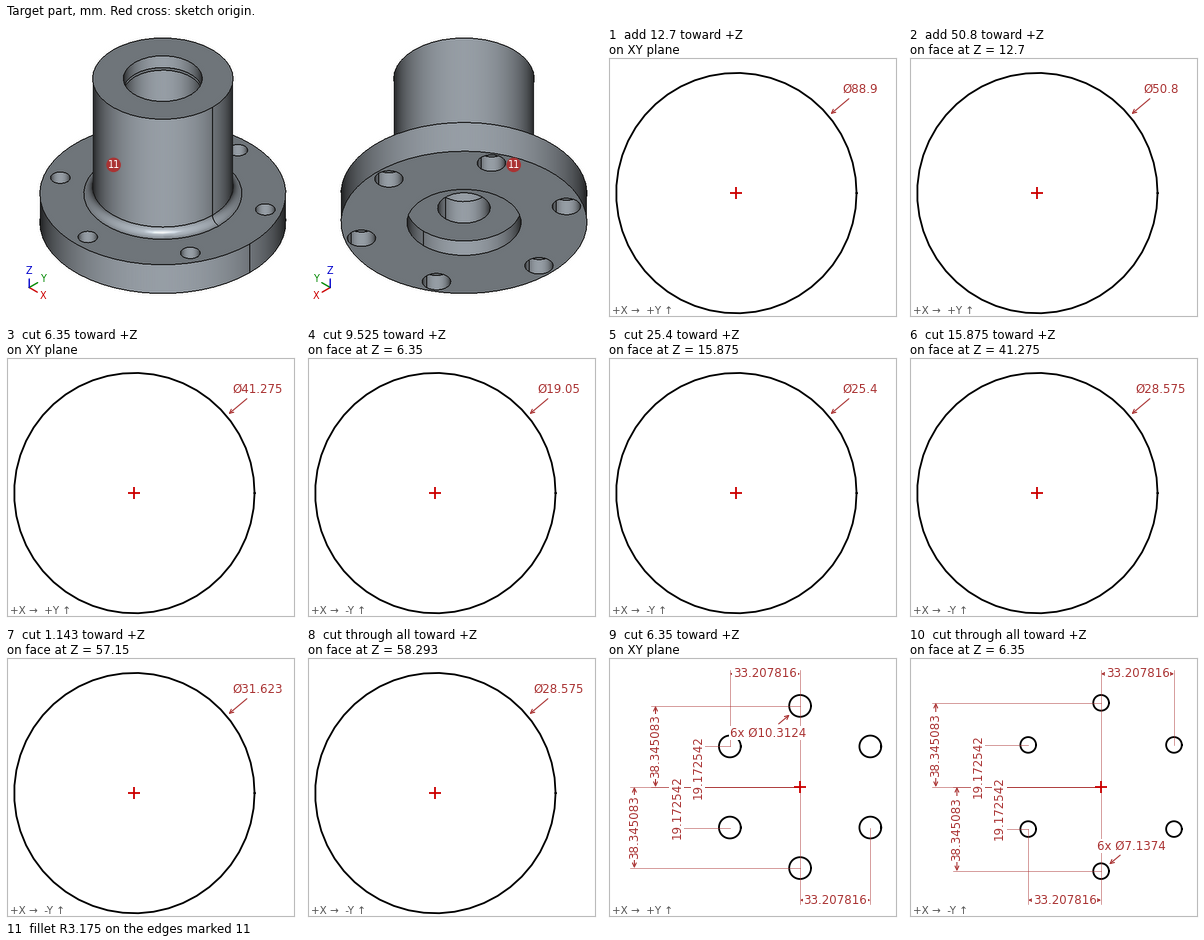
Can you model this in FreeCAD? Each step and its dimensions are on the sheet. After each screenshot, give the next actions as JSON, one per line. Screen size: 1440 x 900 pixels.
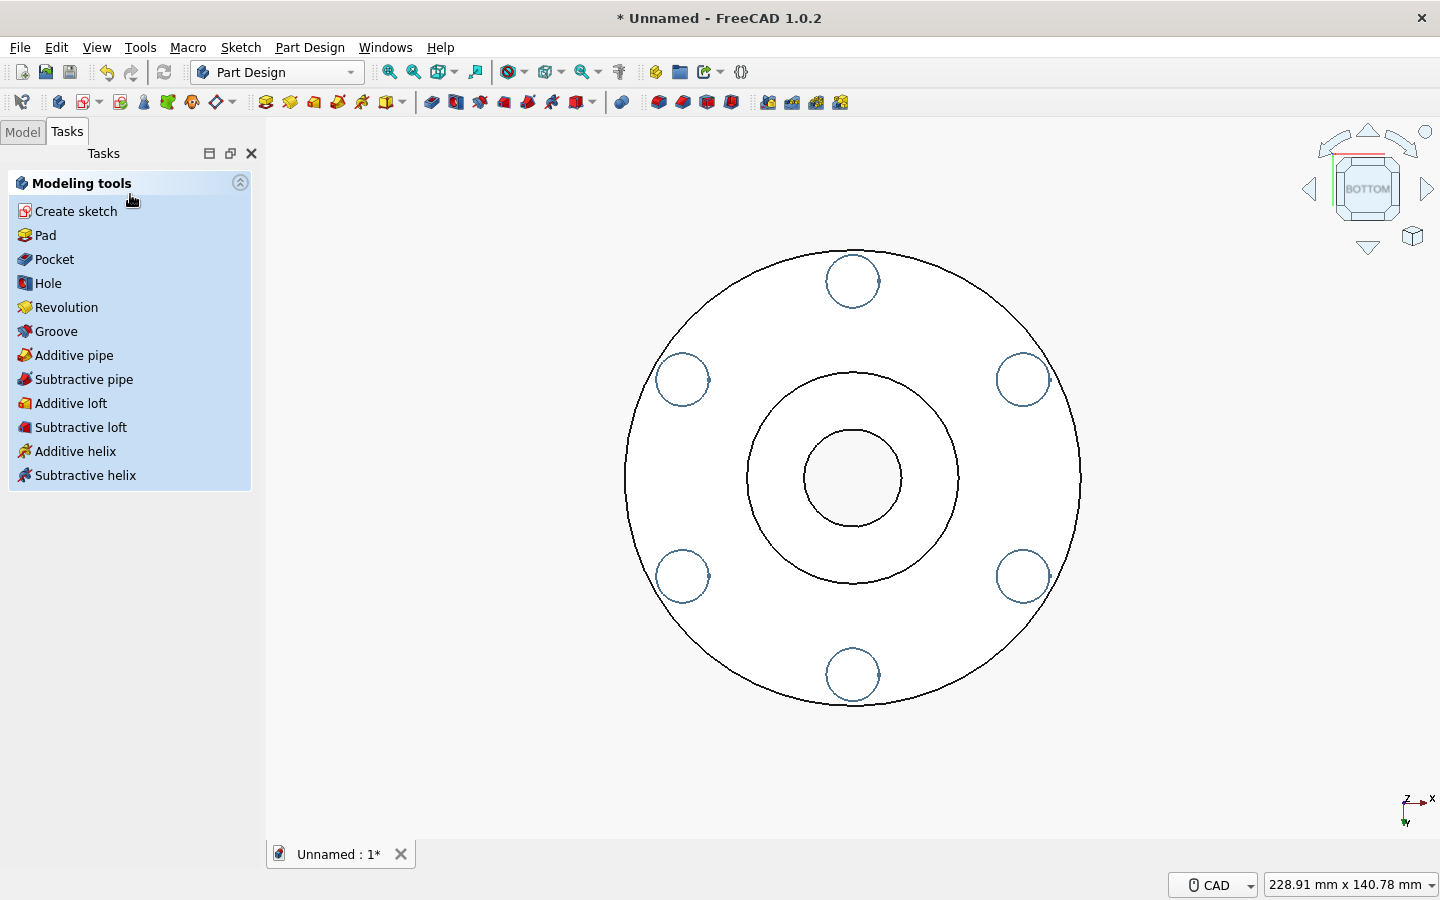
{"action": "left_click", "coordinate": [432, 102]}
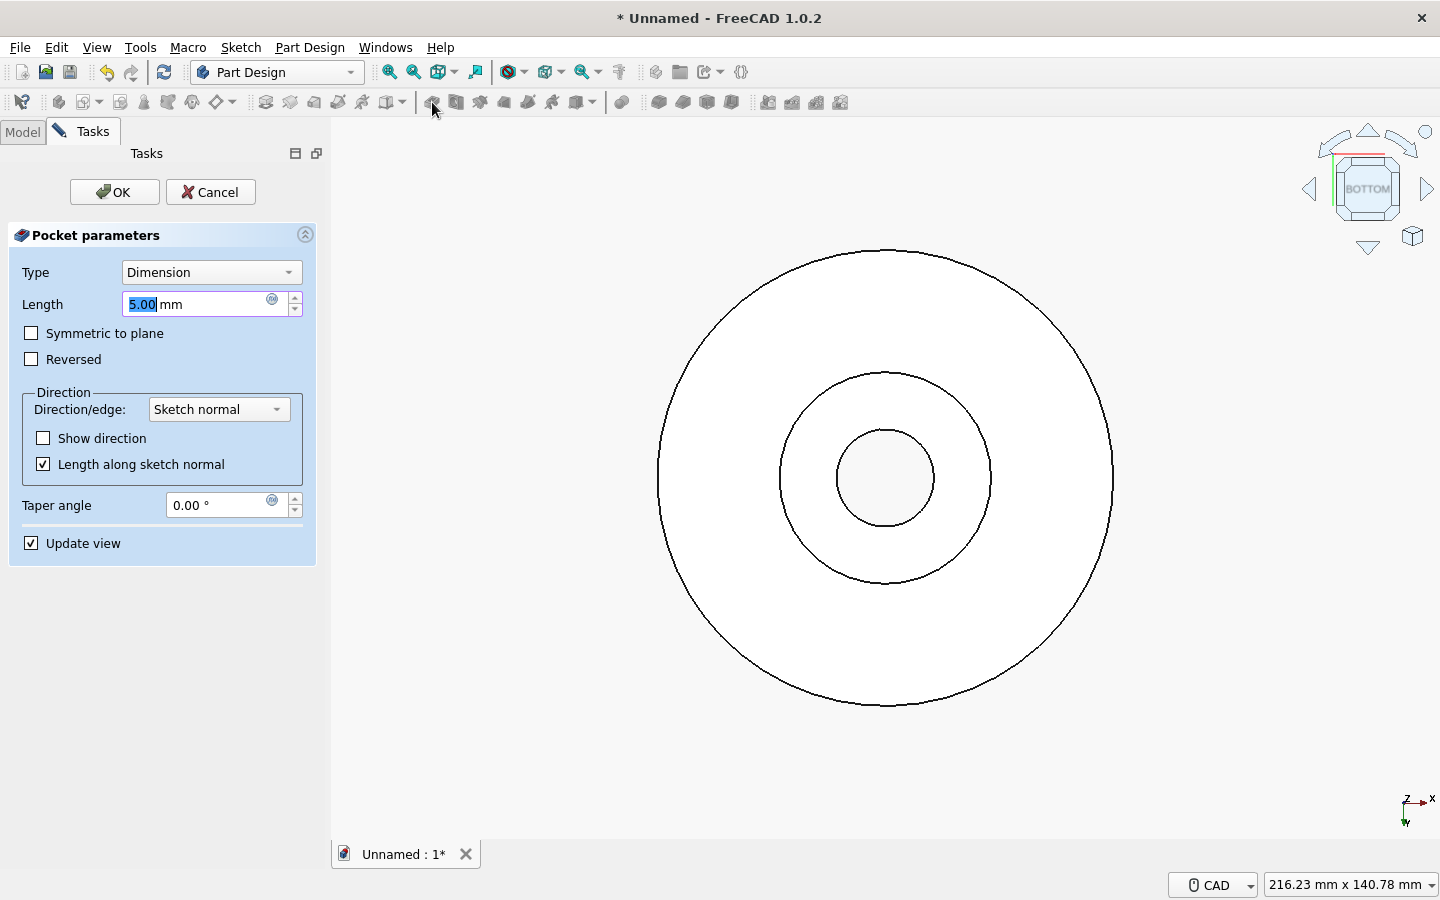
{"action": "type", "text": "6.35"}
{"action": "key", "text": "Tab"}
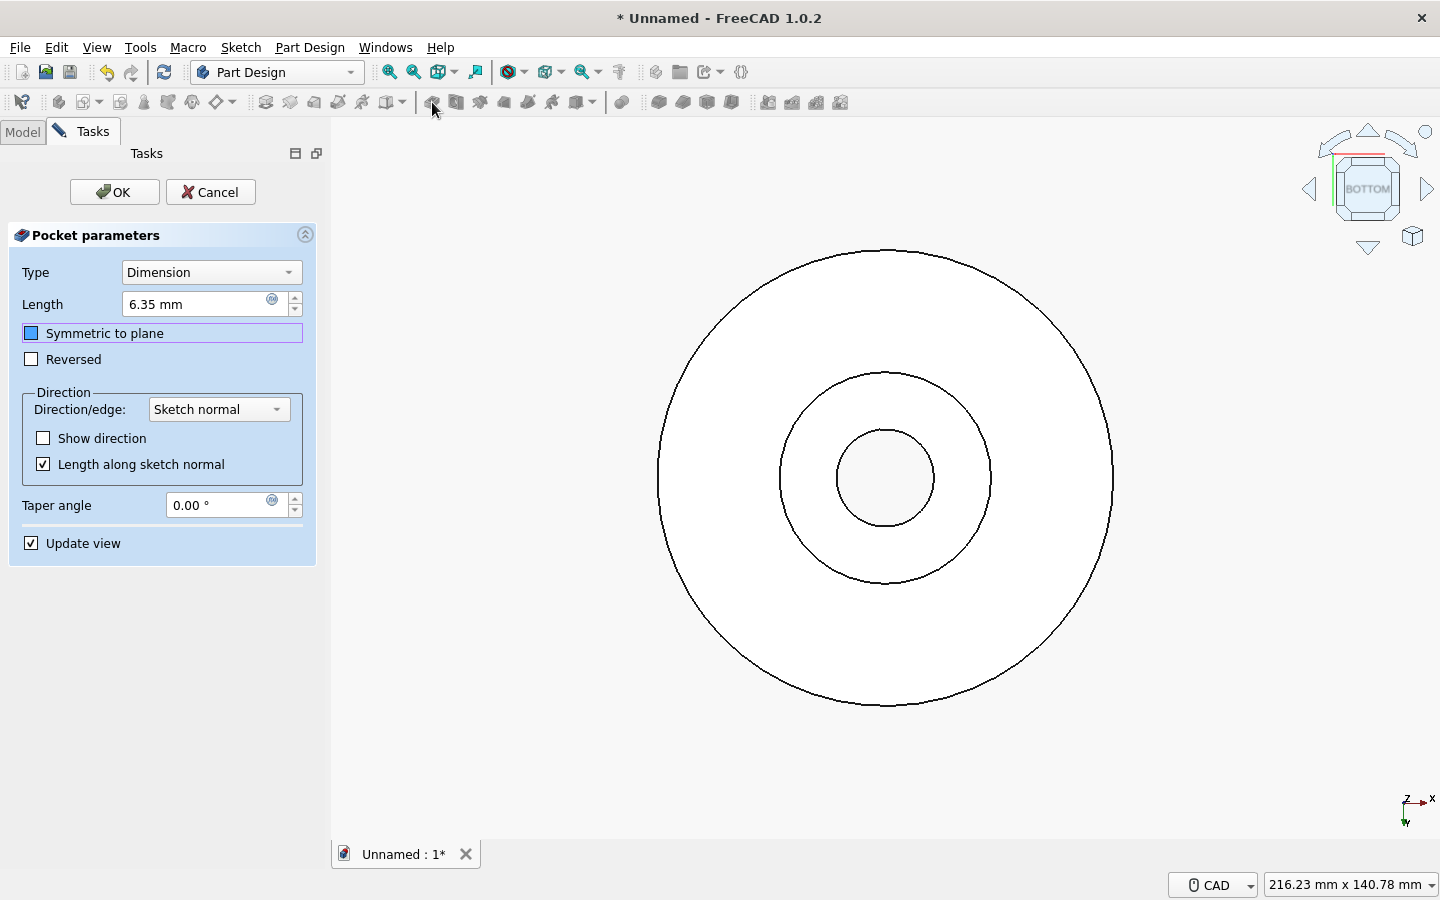
{"action": "left_click", "coordinate": [30, 359]}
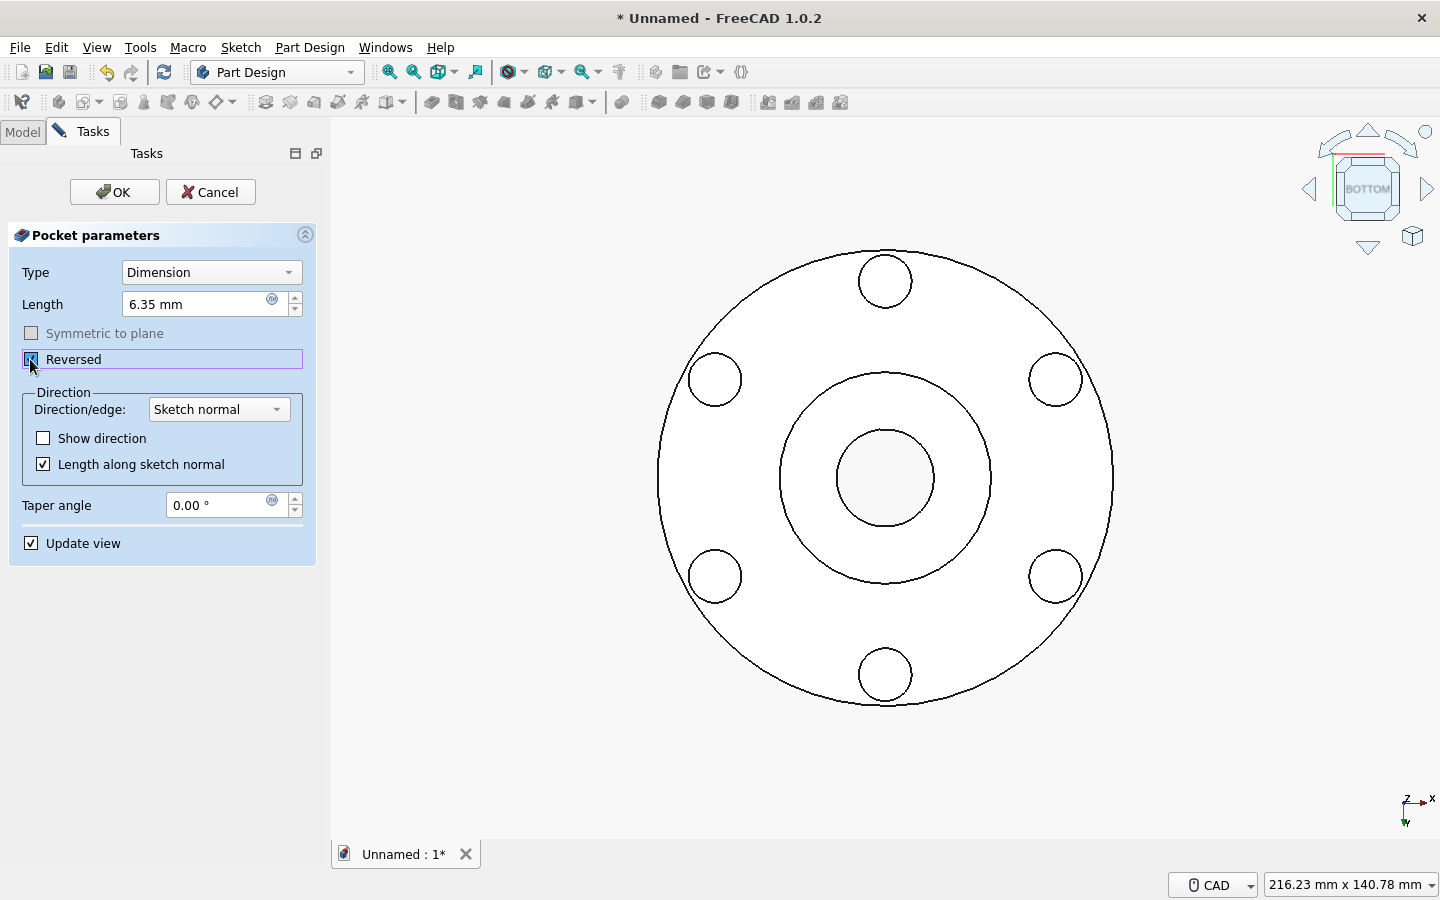
{"action": "left_click", "coordinate": [115, 192]}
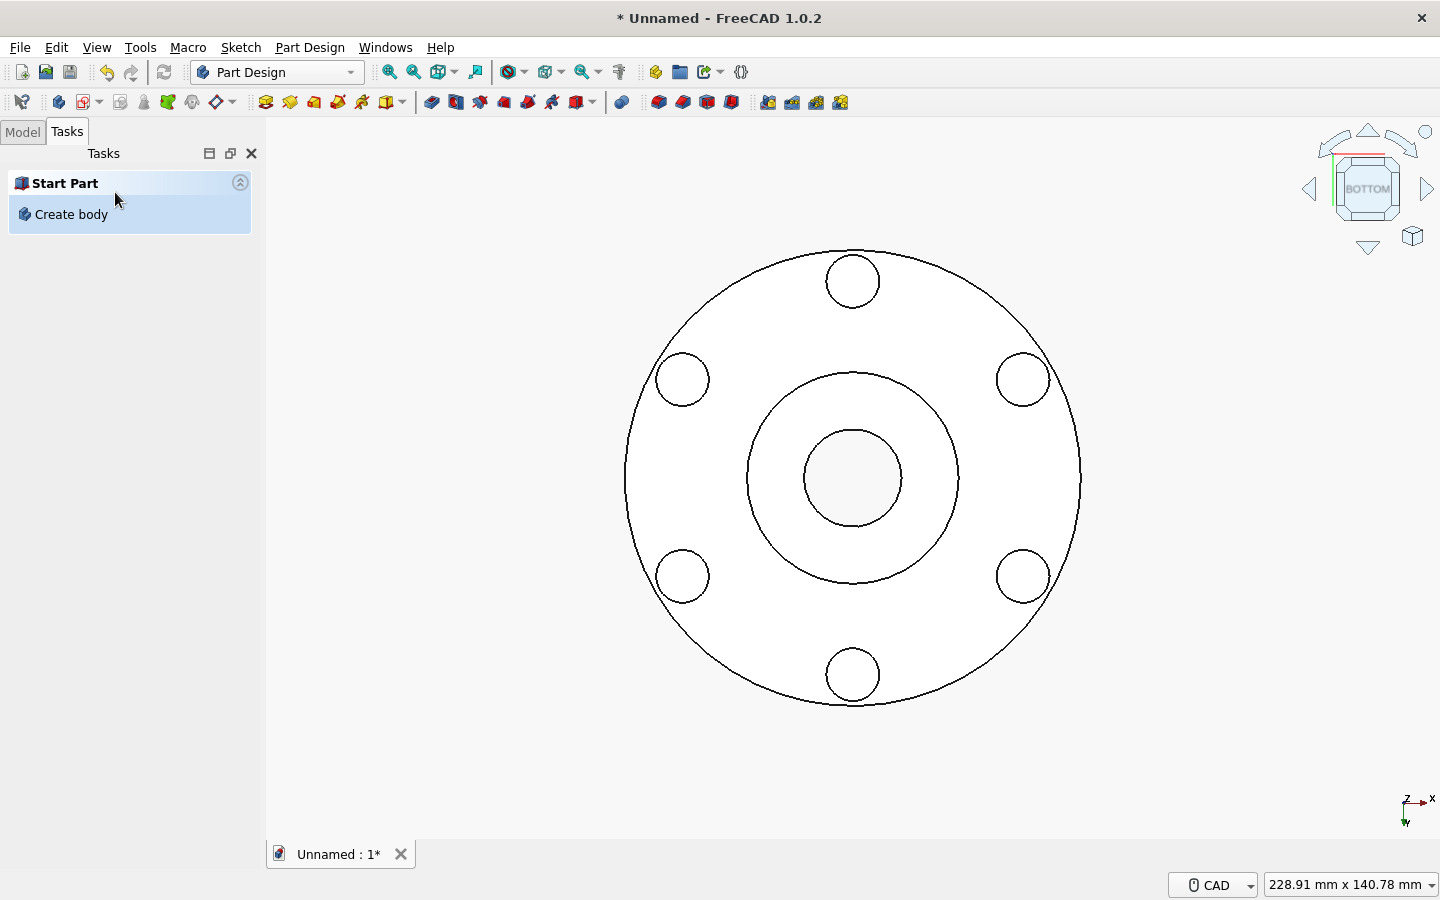
{"action": "left_click", "coordinate": [913, 537]}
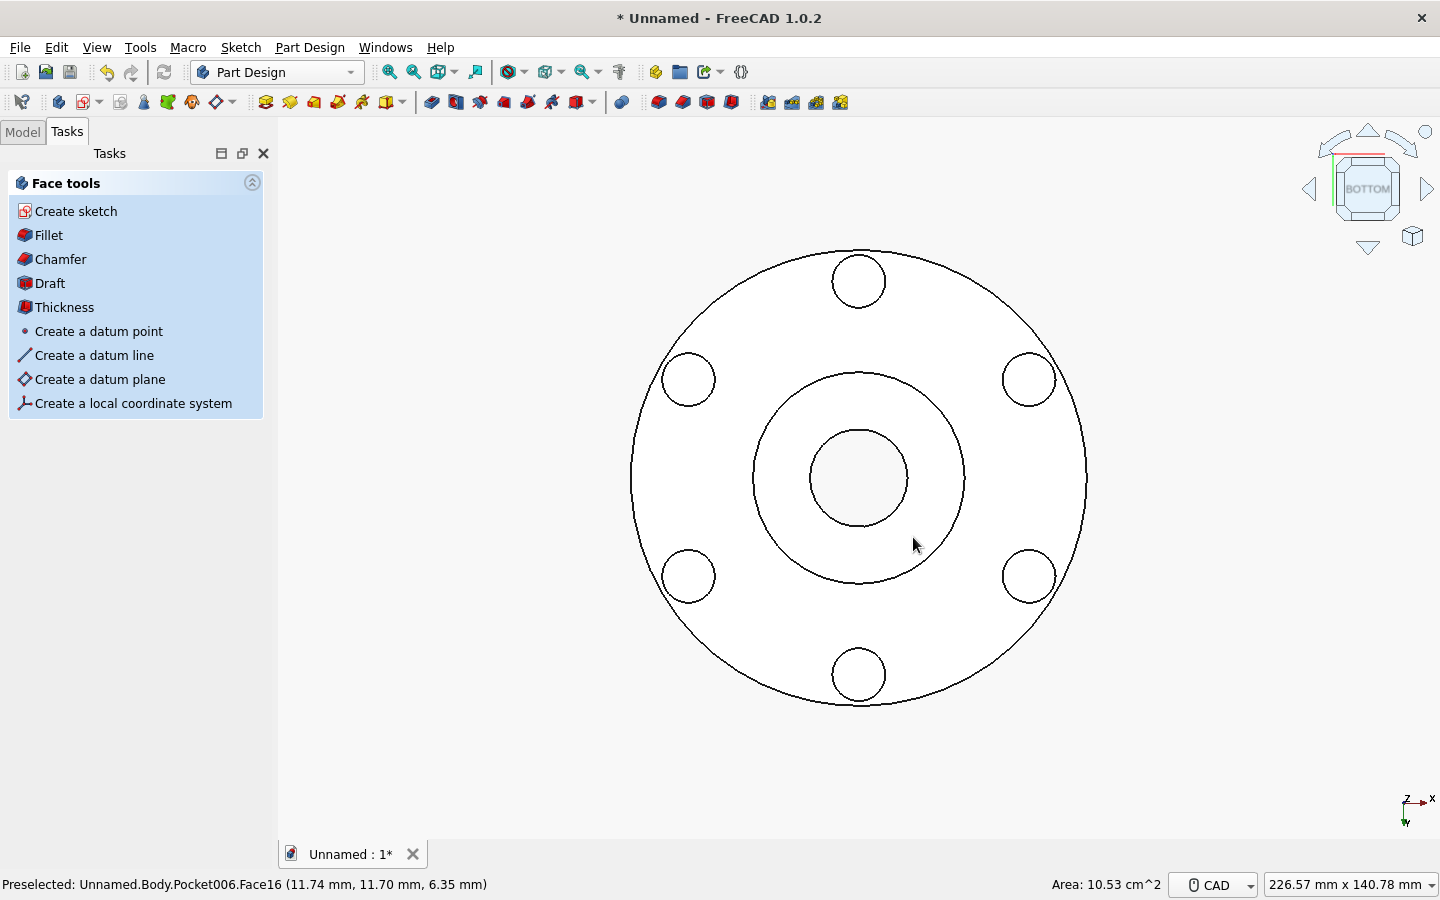
{"action": "left_click", "coordinate": [84, 102]}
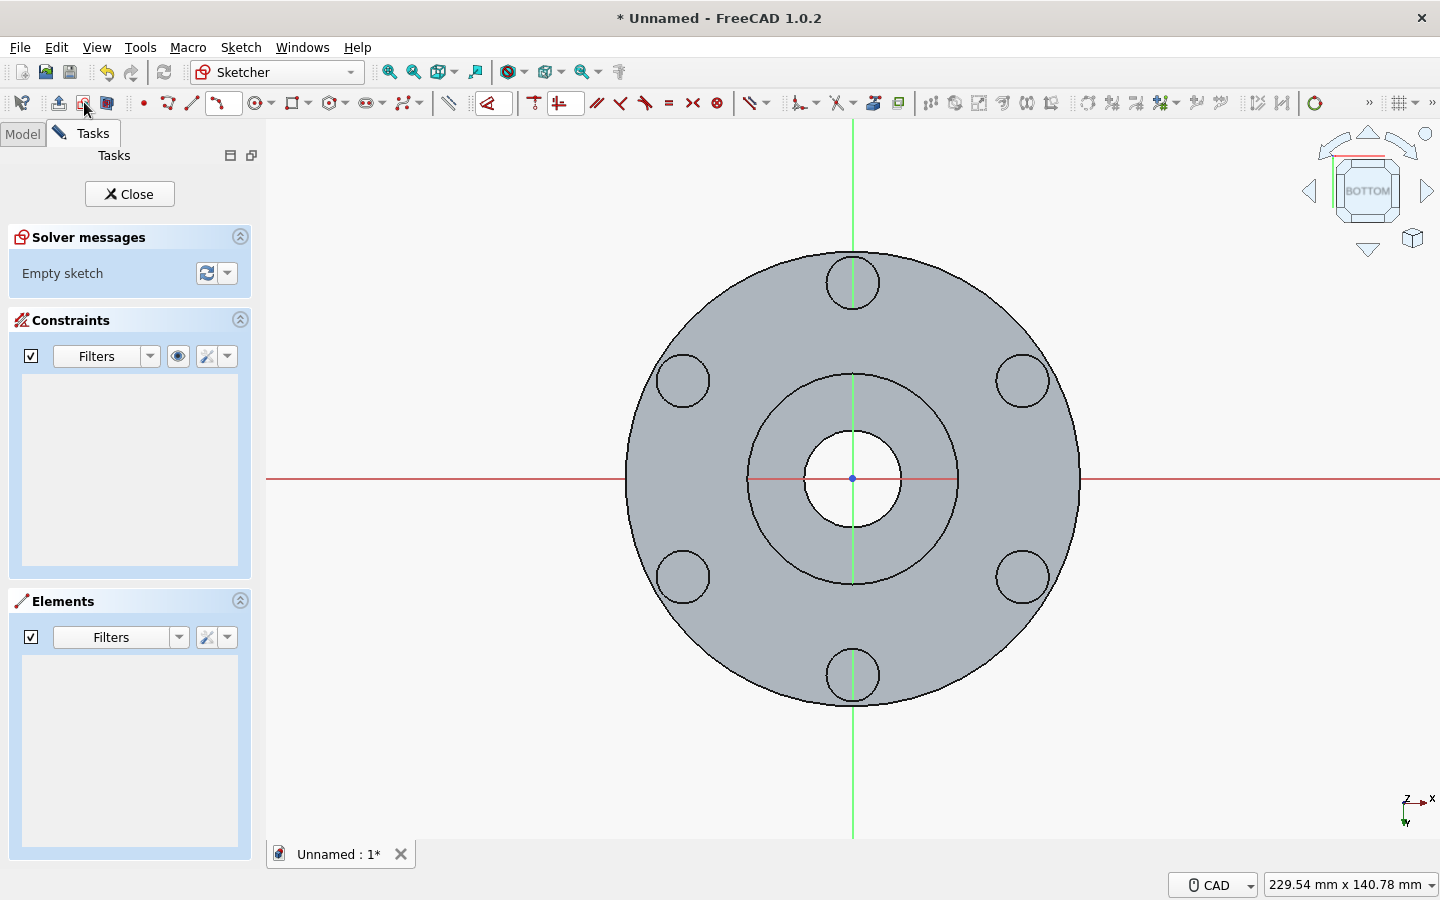
{"action": "key", "text": "g c"}